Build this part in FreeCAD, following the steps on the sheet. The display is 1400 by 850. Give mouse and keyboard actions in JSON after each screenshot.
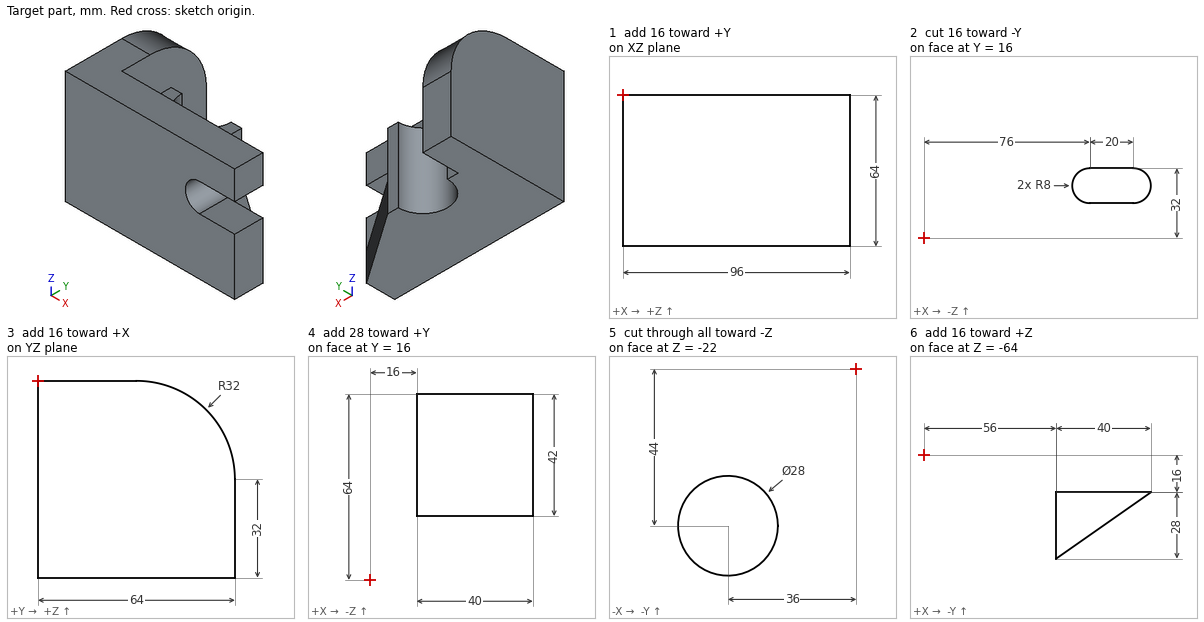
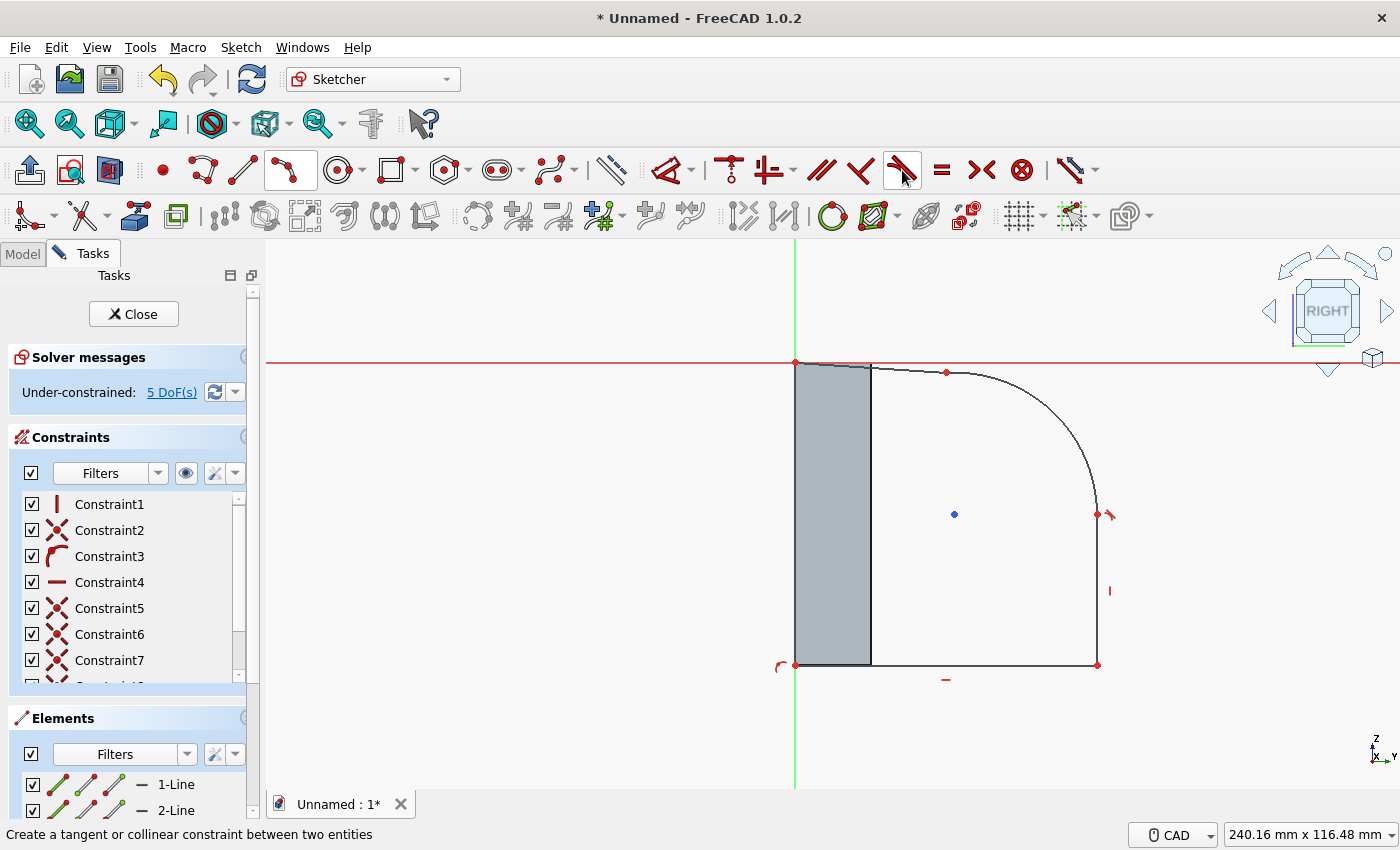
{"action": "left_click", "coordinate": [840, 366]}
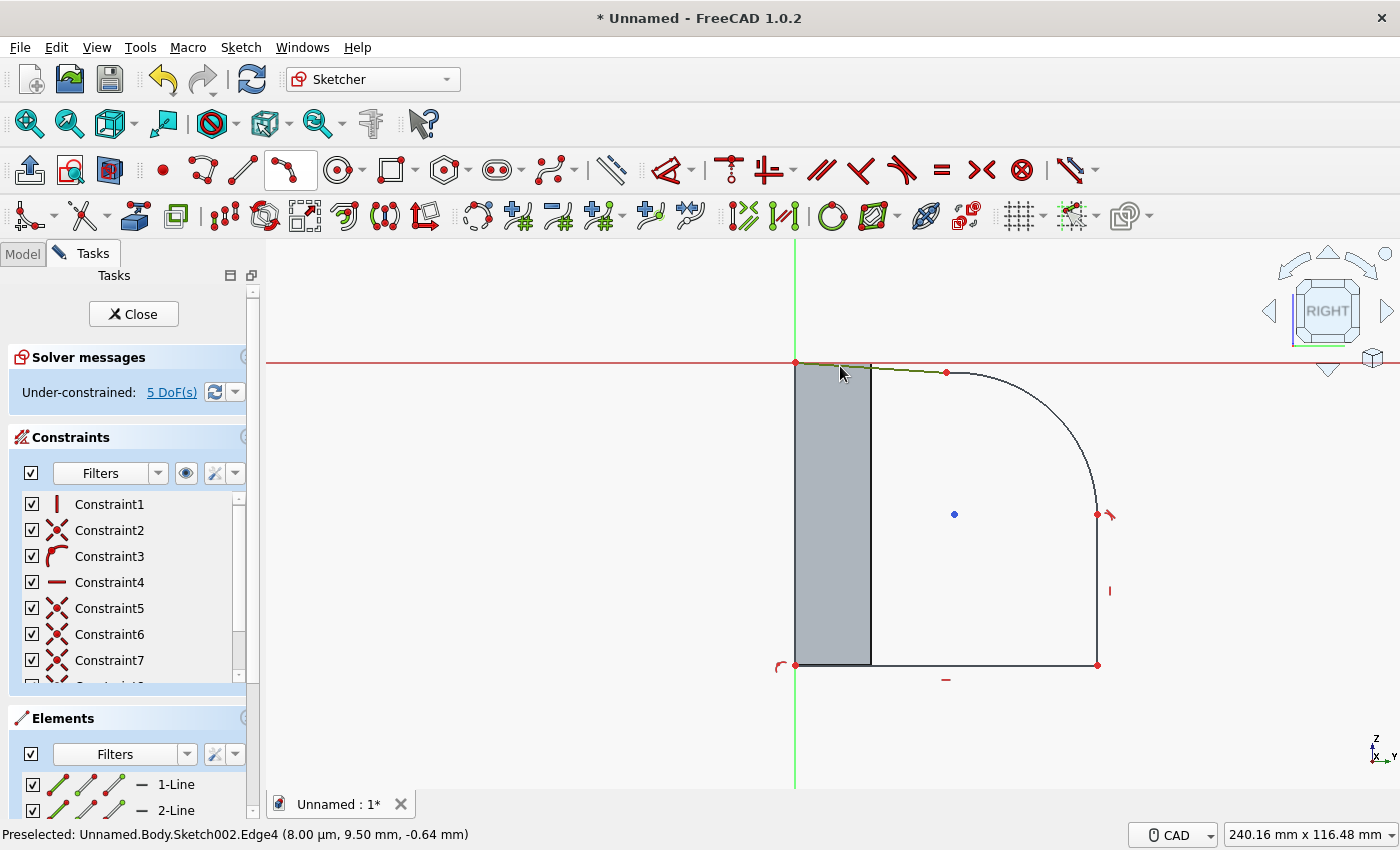
{"action": "left_click", "coordinate": [1080, 448]}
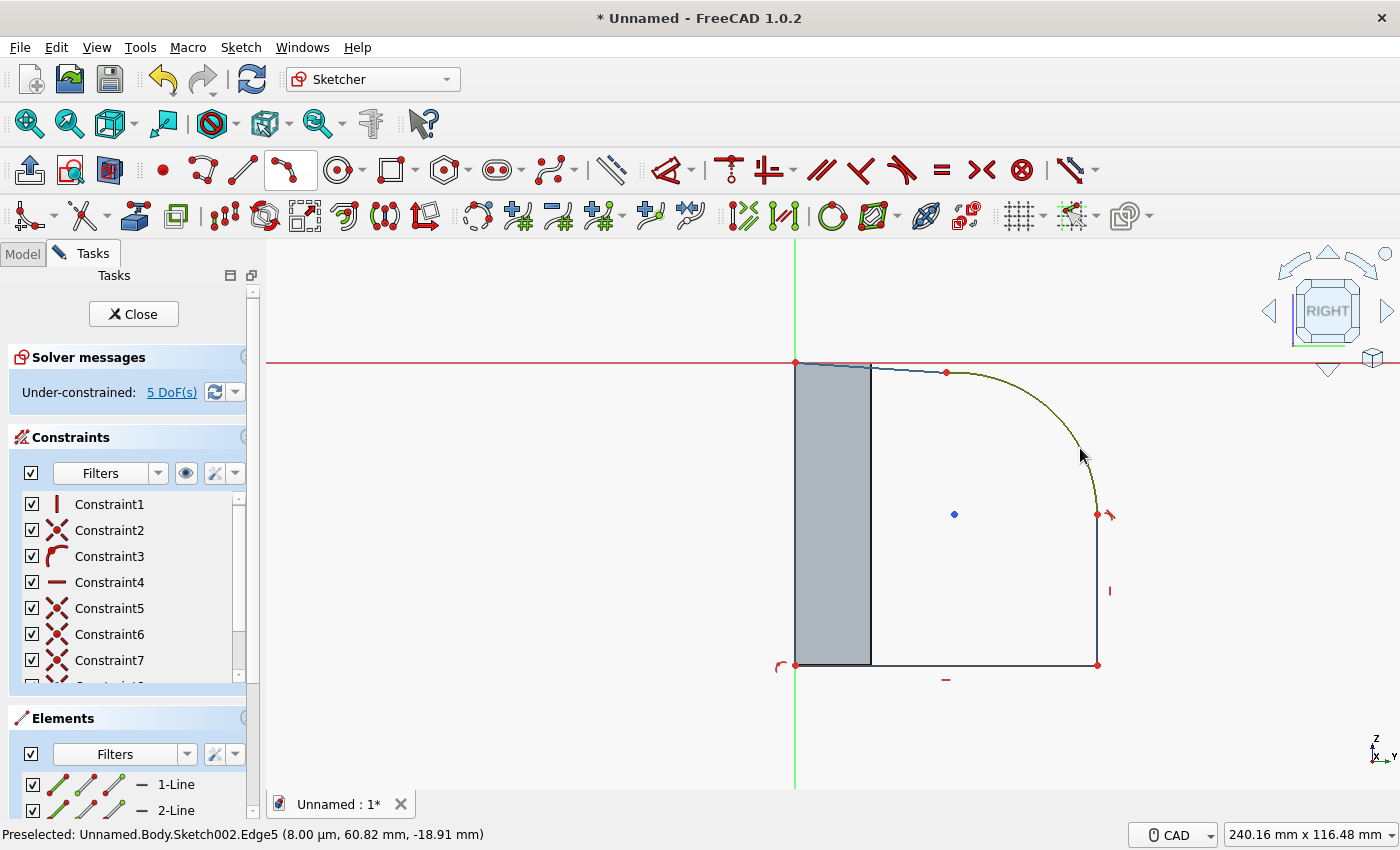
{"action": "key", "text": "t"}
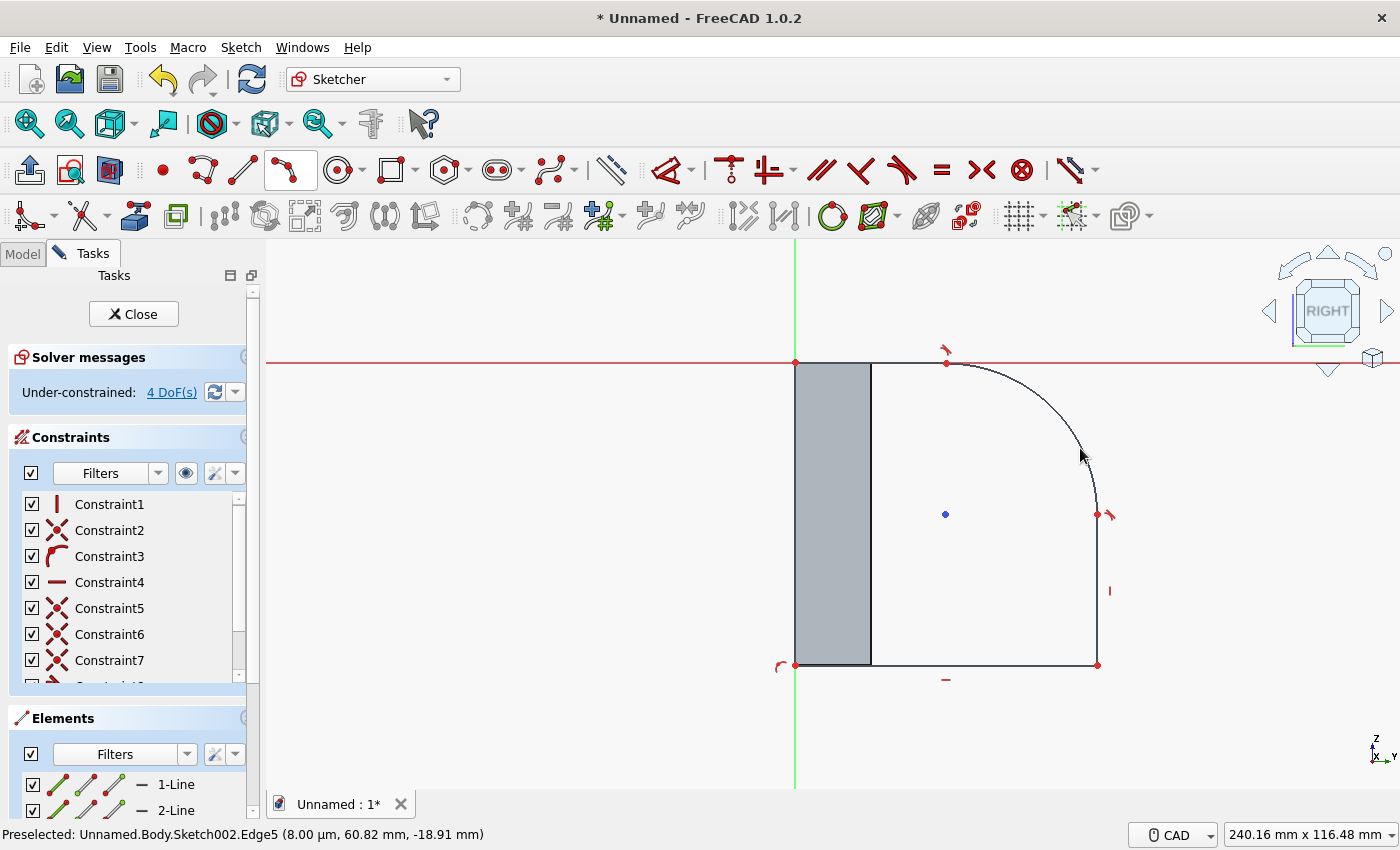
{"action": "left_click", "coordinate": [841, 363]}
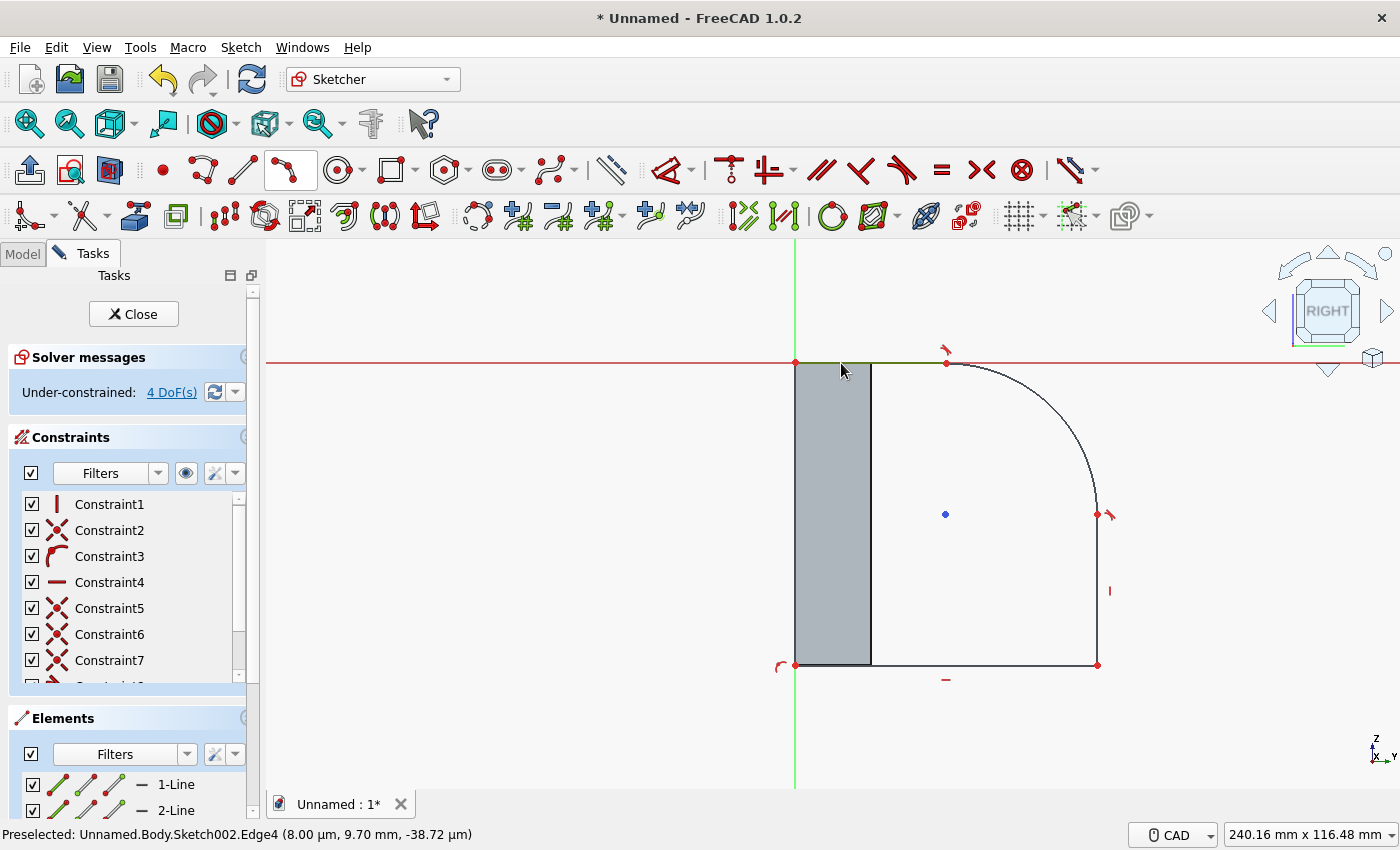
{"action": "key", "text": "h"}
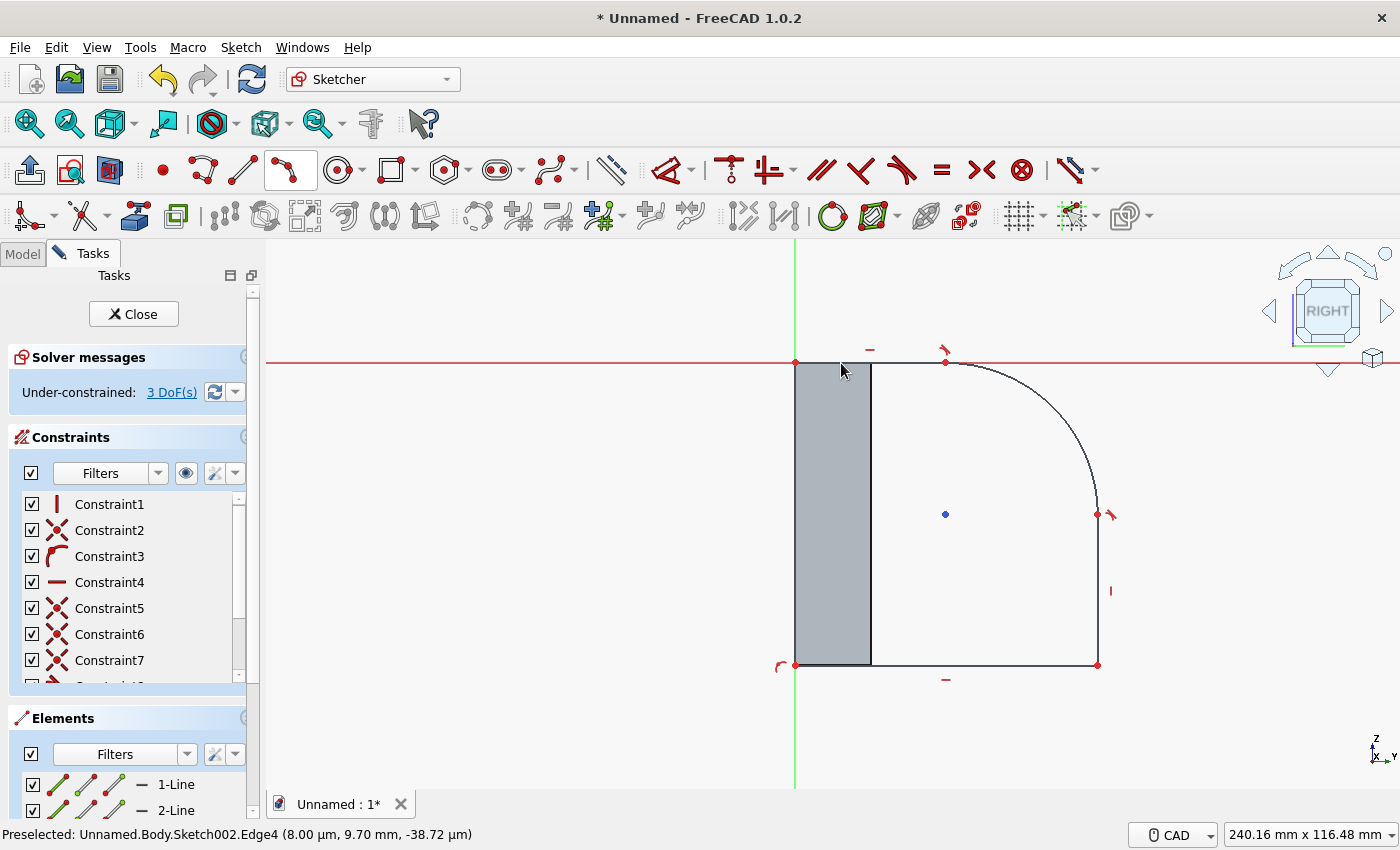
{"action": "left_click", "coordinate": [666, 170]}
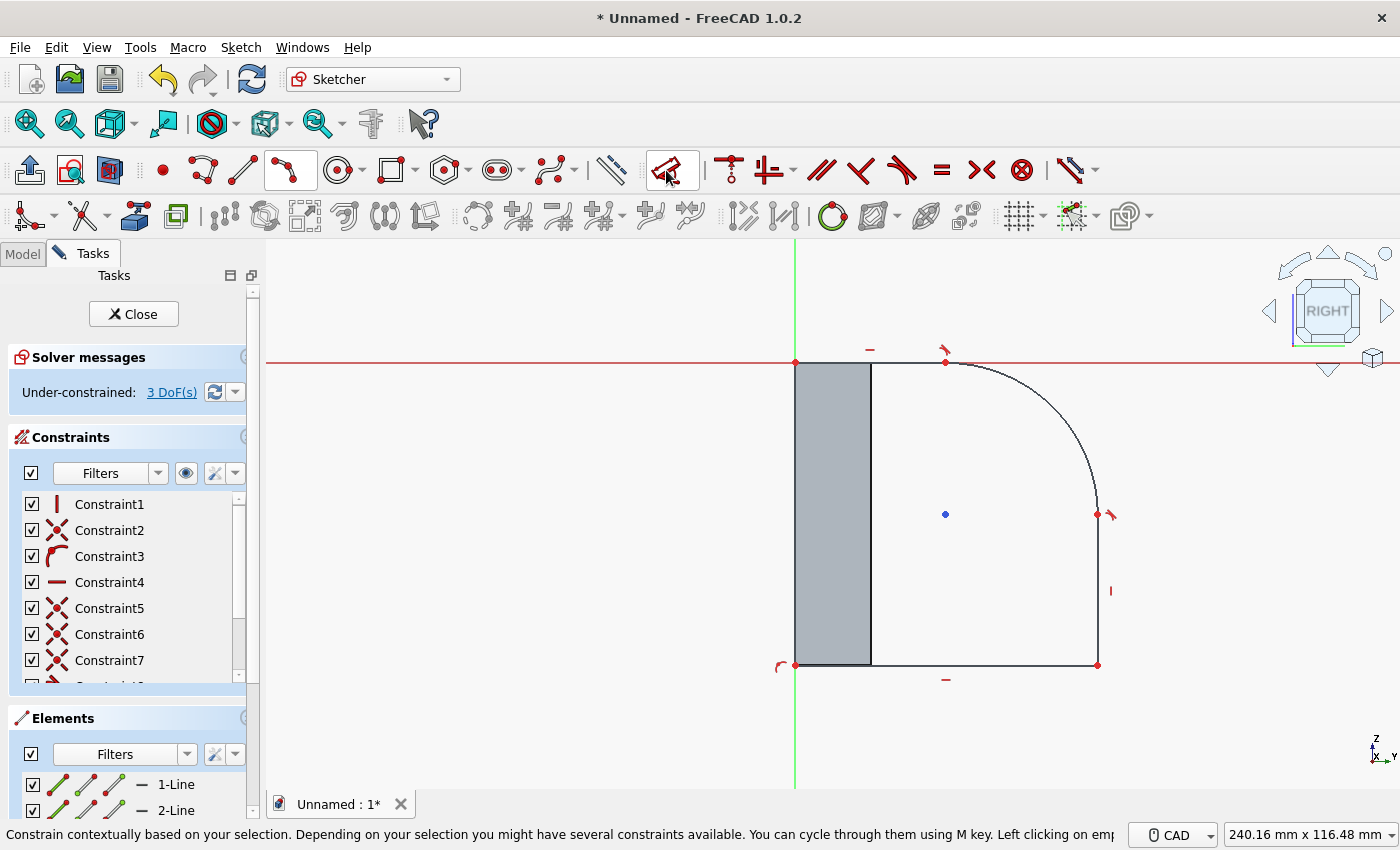
{"action": "left_click", "coordinate": [1081, 446]}
{"action": "left_click", "coordinate": [1110, 431]}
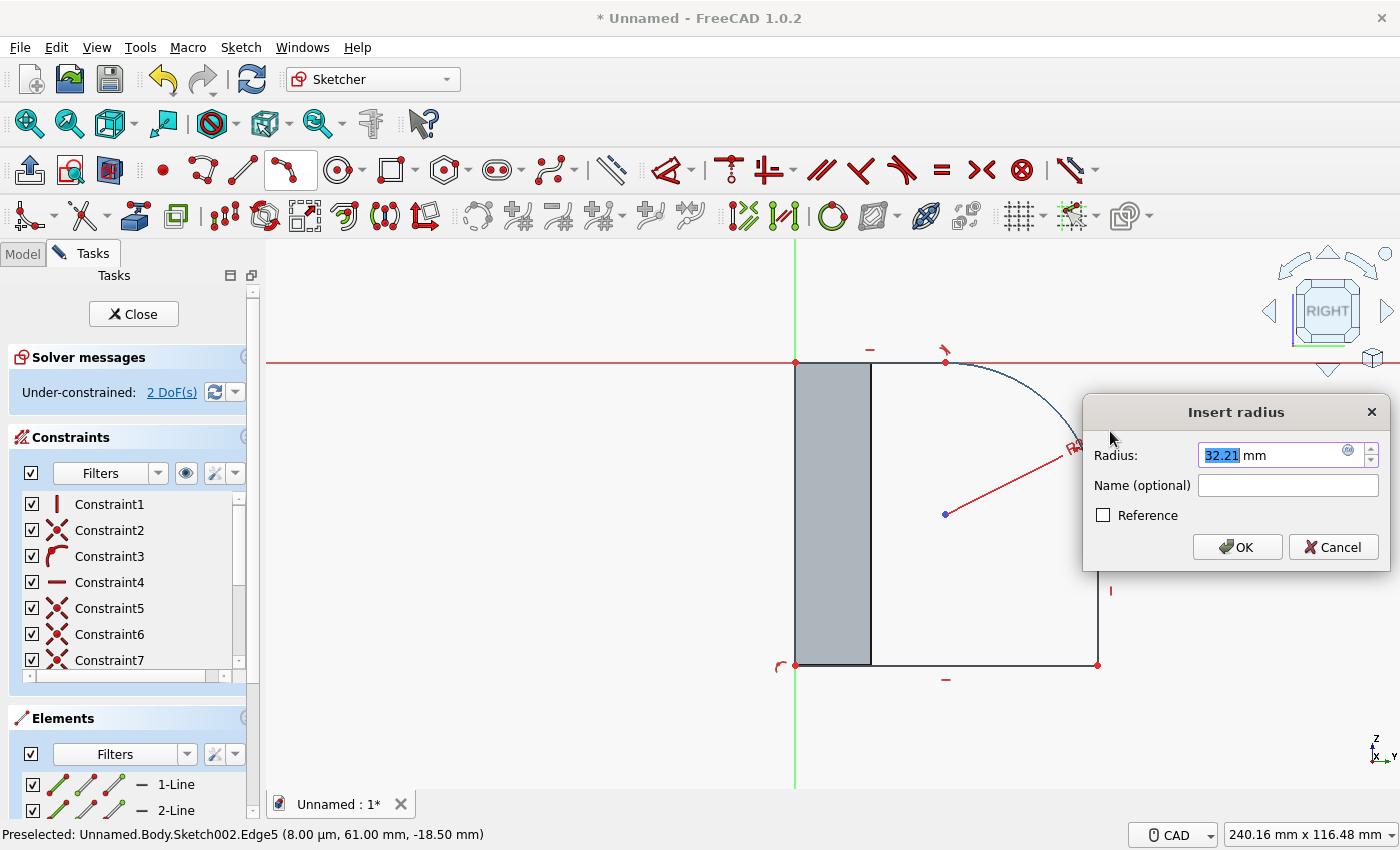
{"action": "type", "text": "32"}
{"action": "key", "text": "Return"}